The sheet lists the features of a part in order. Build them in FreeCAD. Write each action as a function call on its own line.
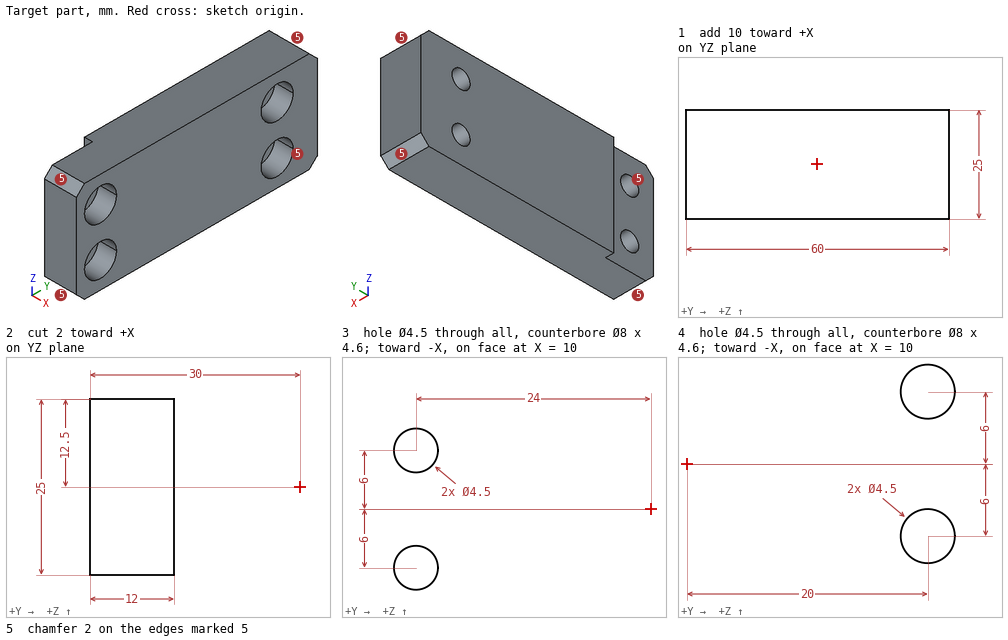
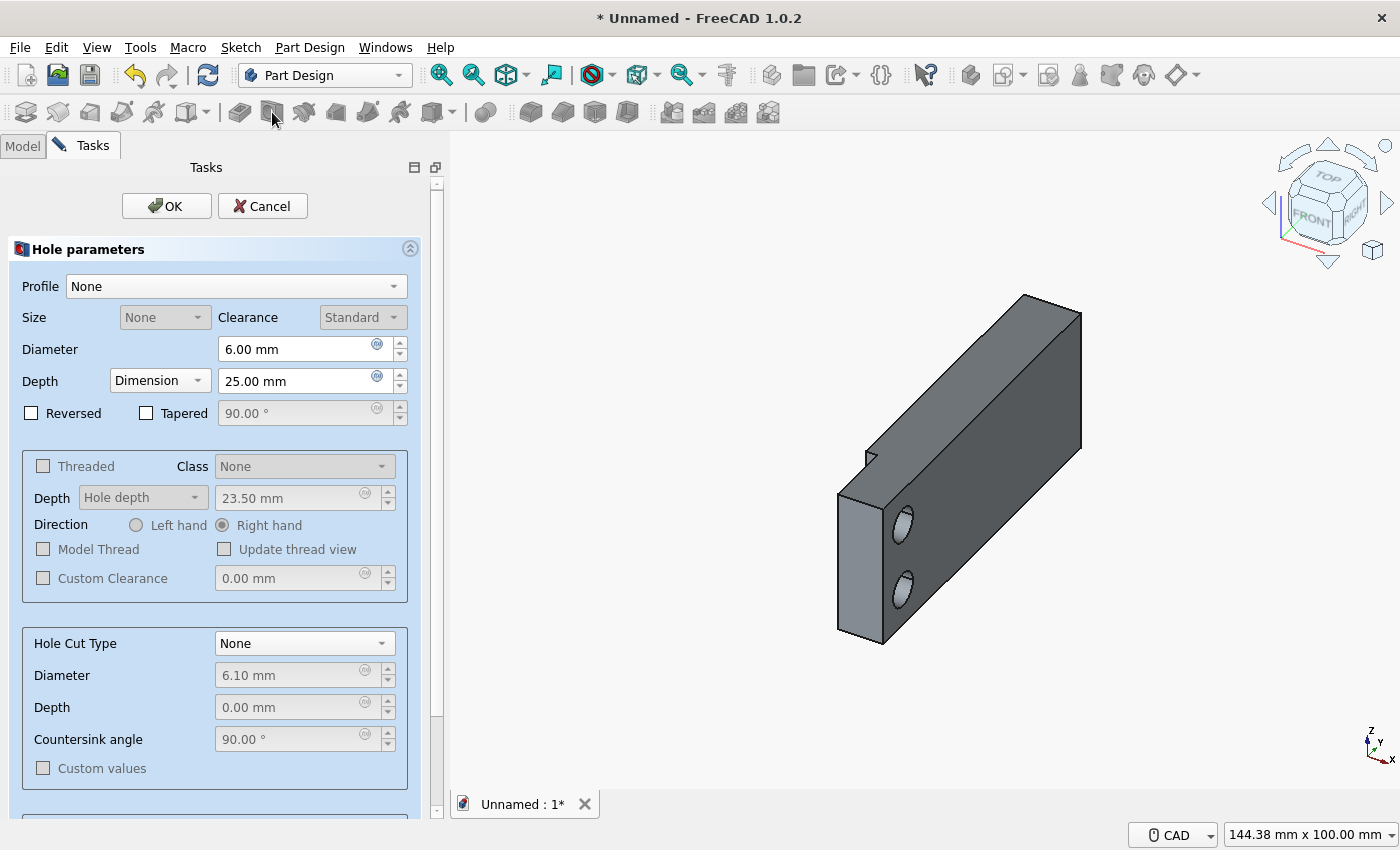
triple_click(305, 349)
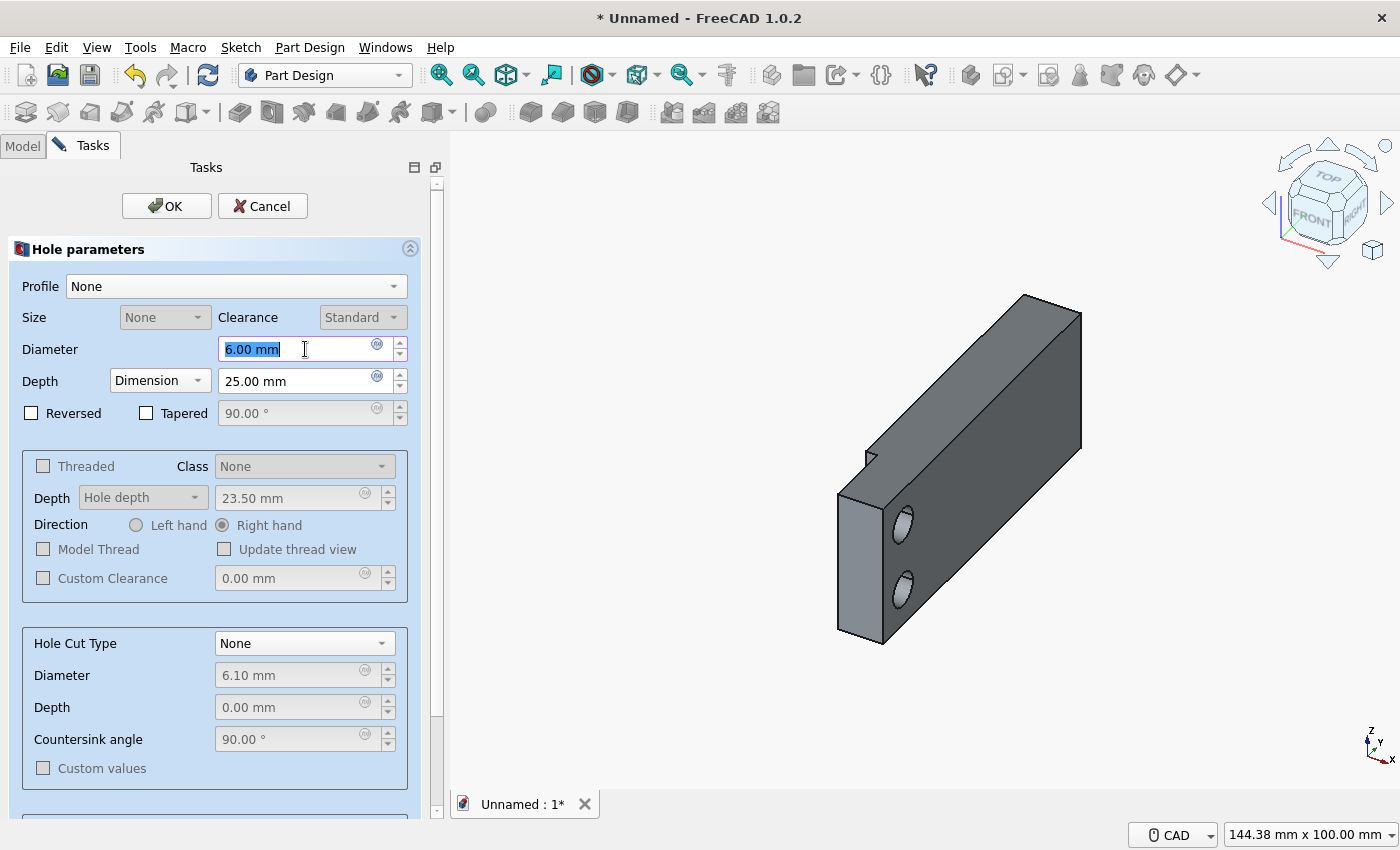
text(4.5)
key(Tab)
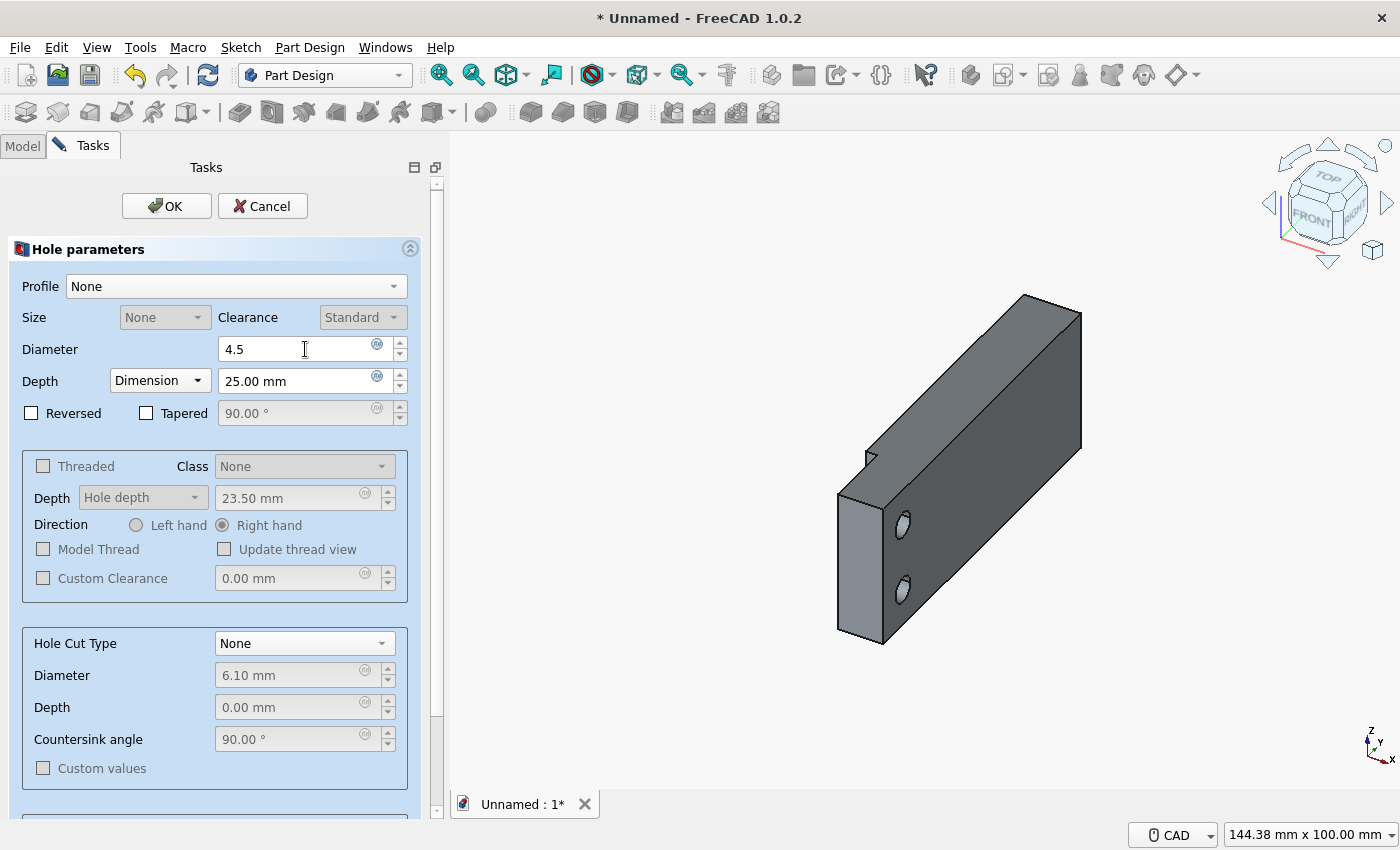
click(161, 380)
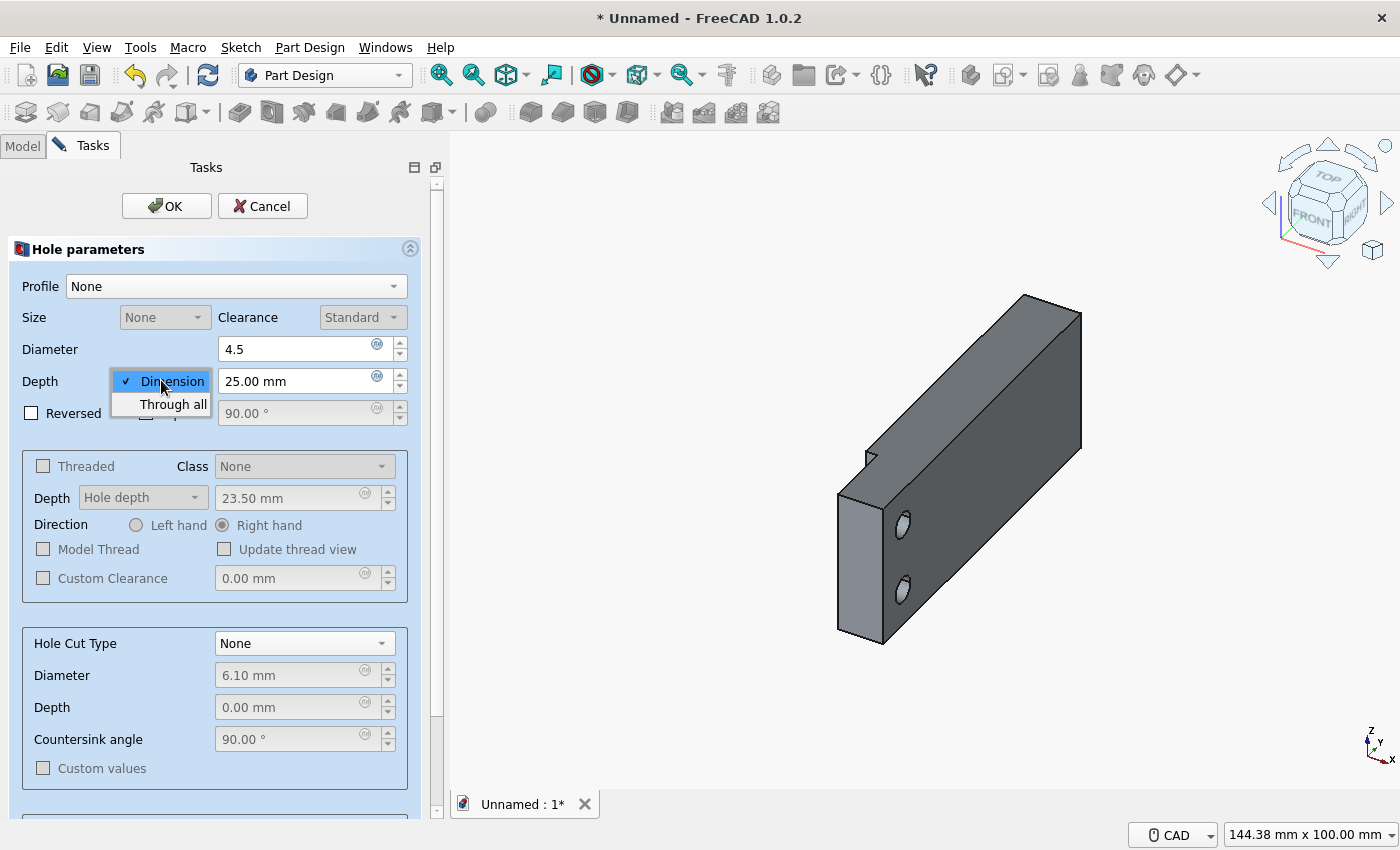
click(160, 404)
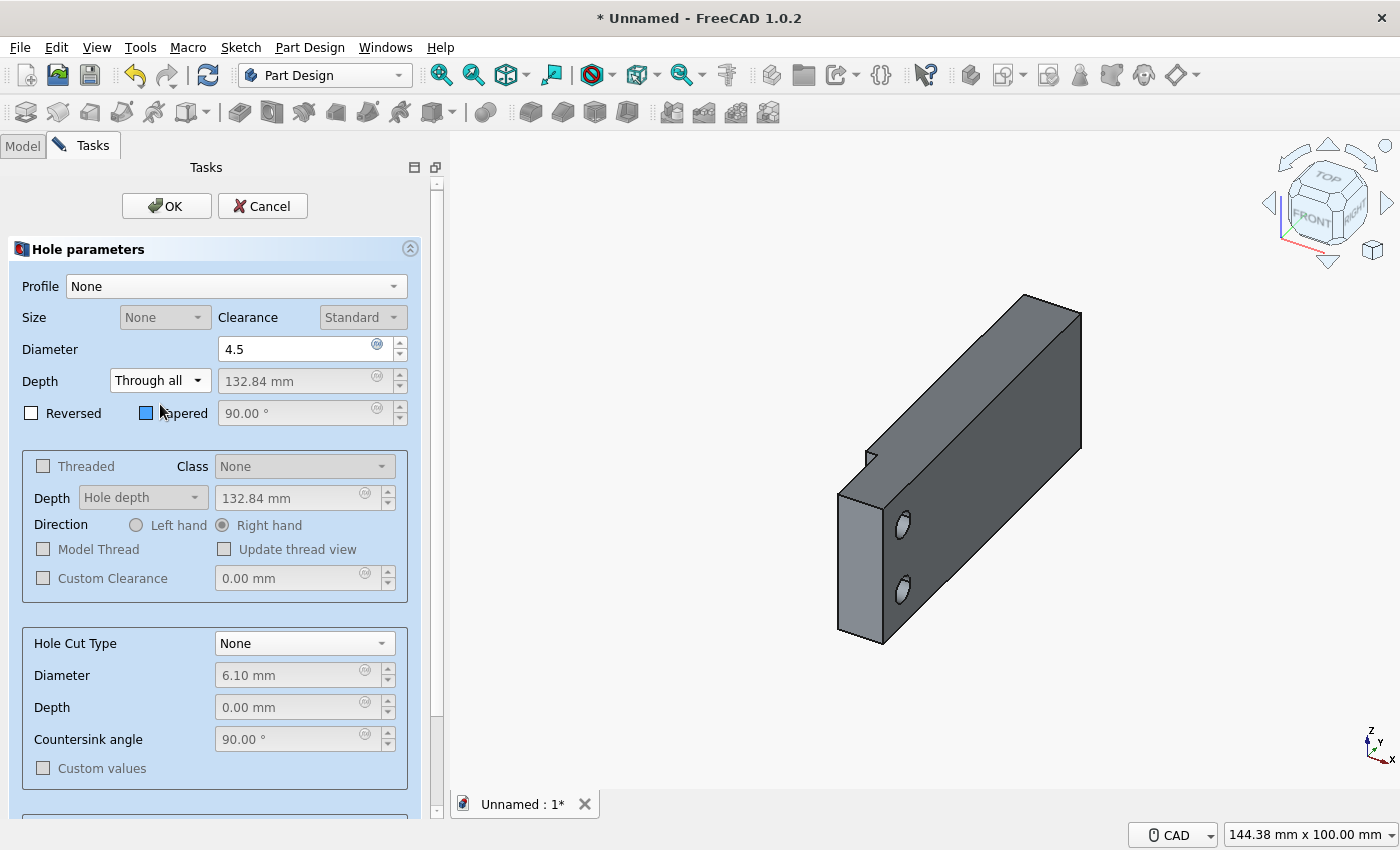
click(306, 644)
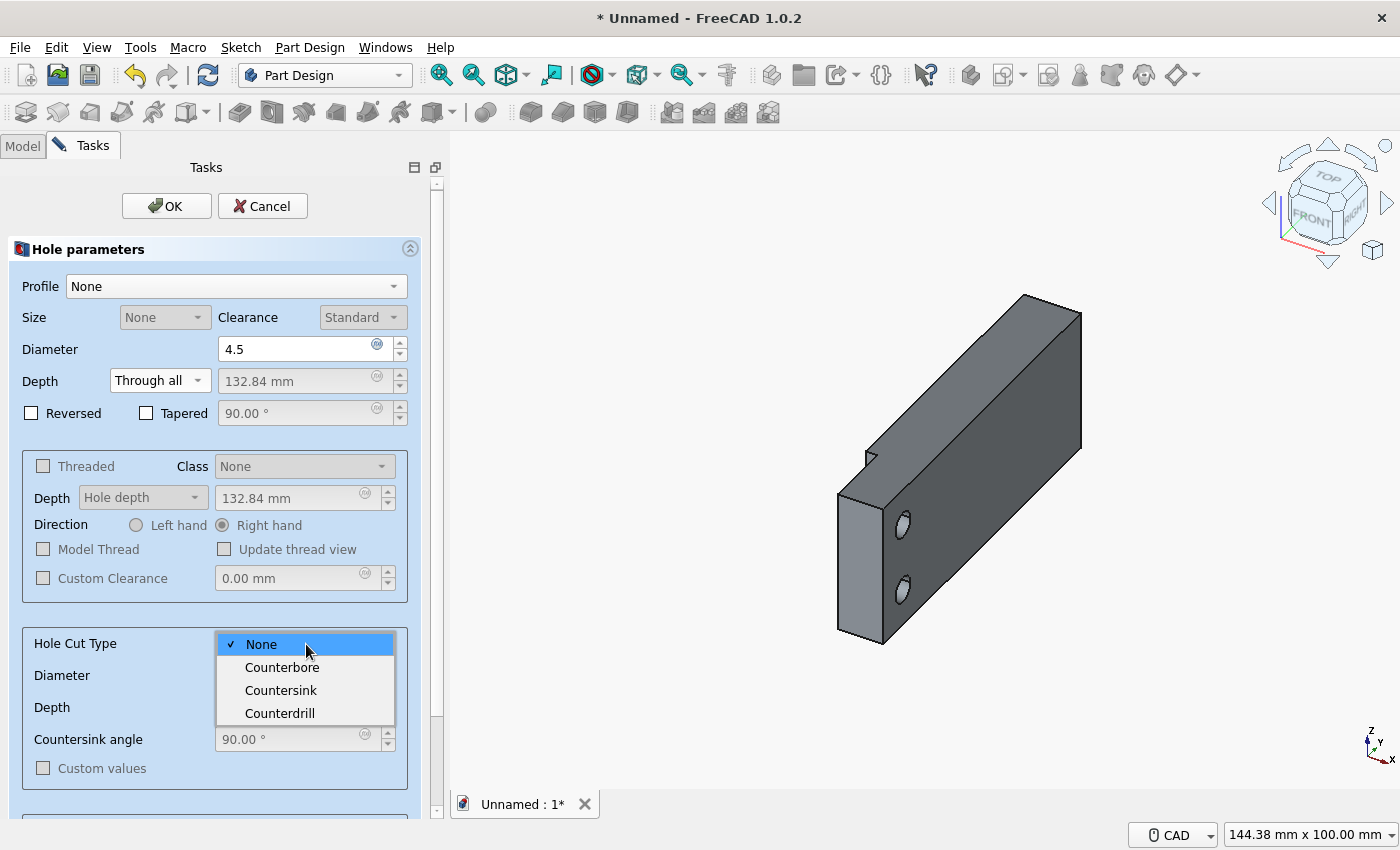
click(304, 668)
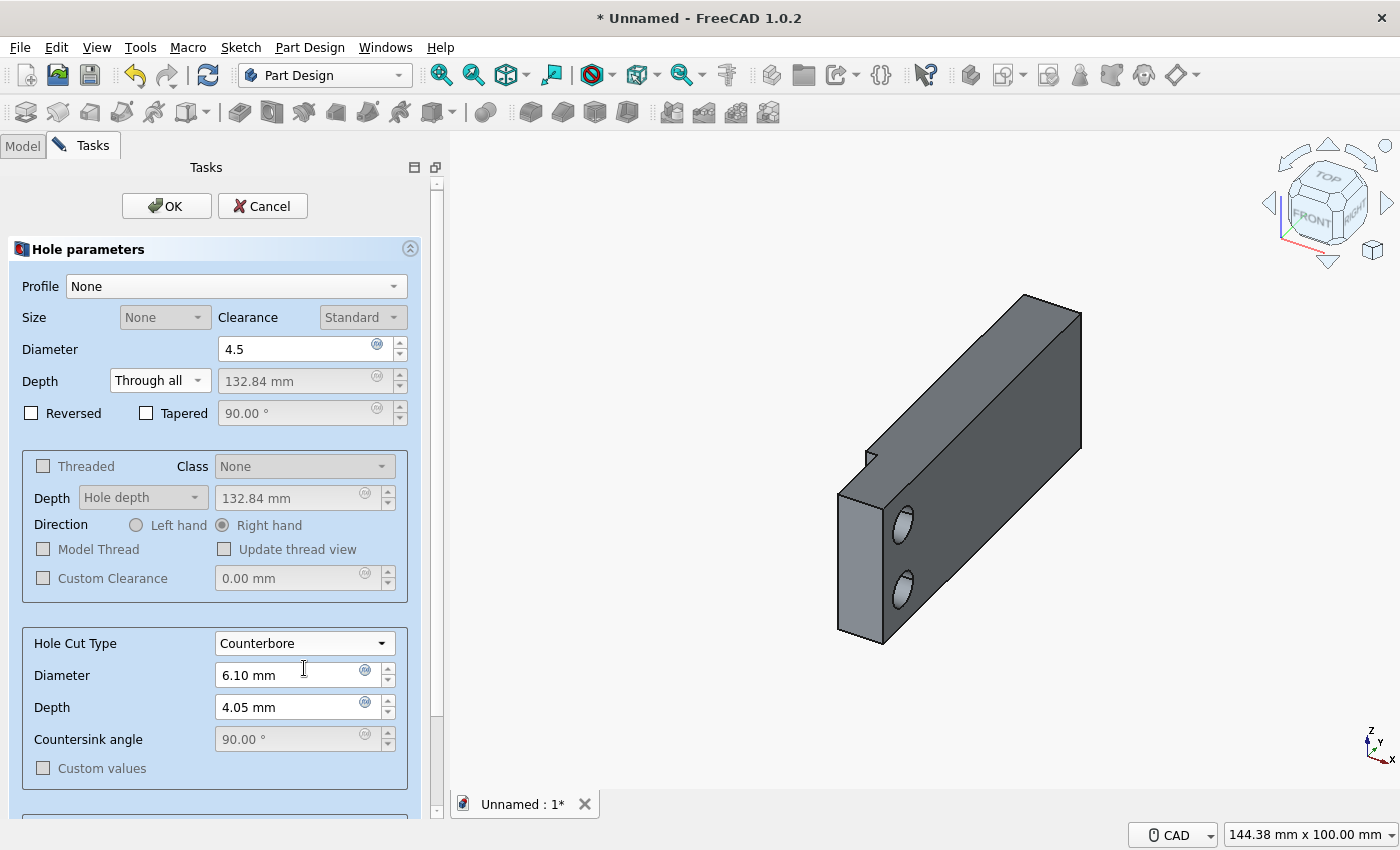
triple_click(298, 675)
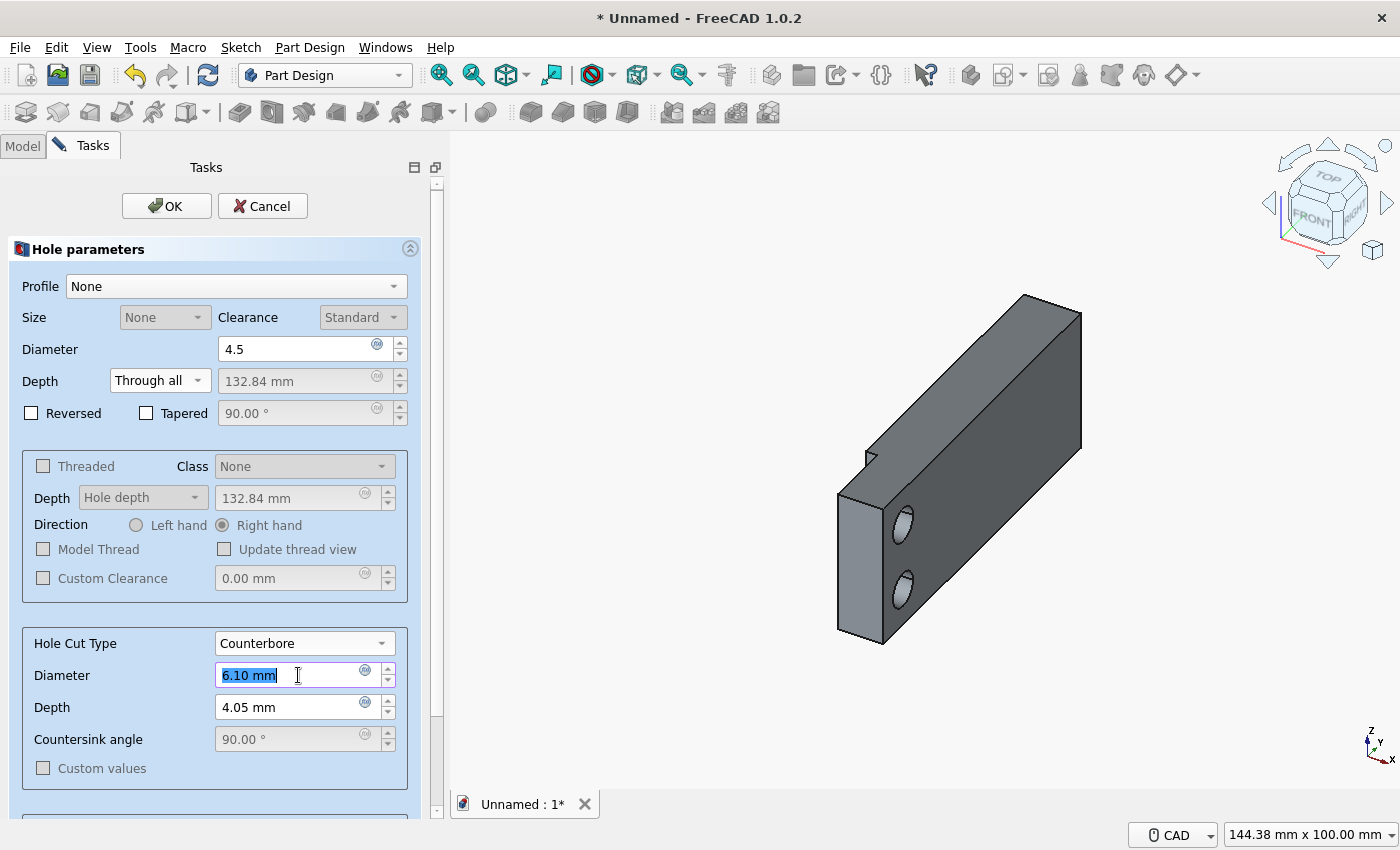
text(8)
key(Tab)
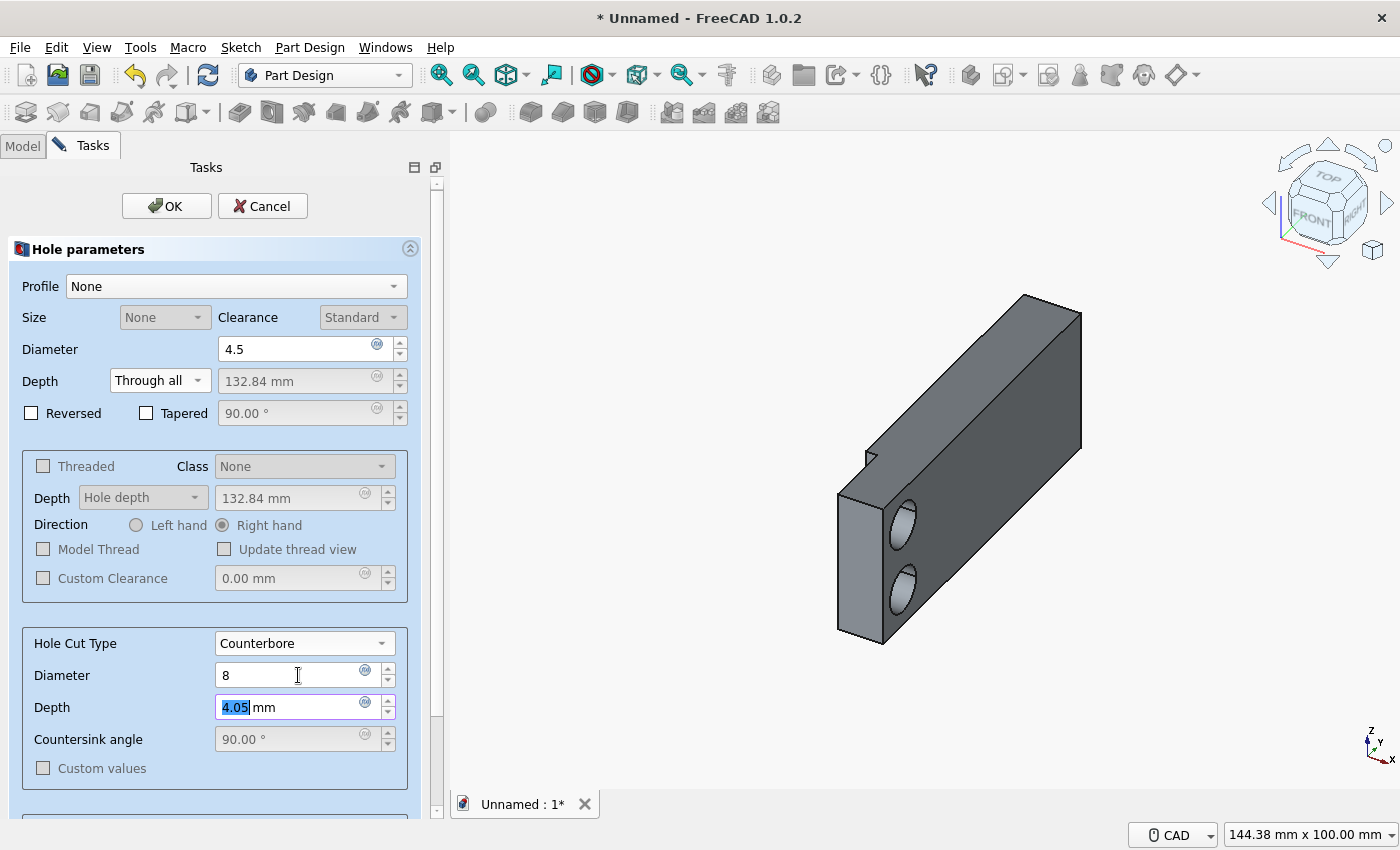
text(4.6)
key(Tab)